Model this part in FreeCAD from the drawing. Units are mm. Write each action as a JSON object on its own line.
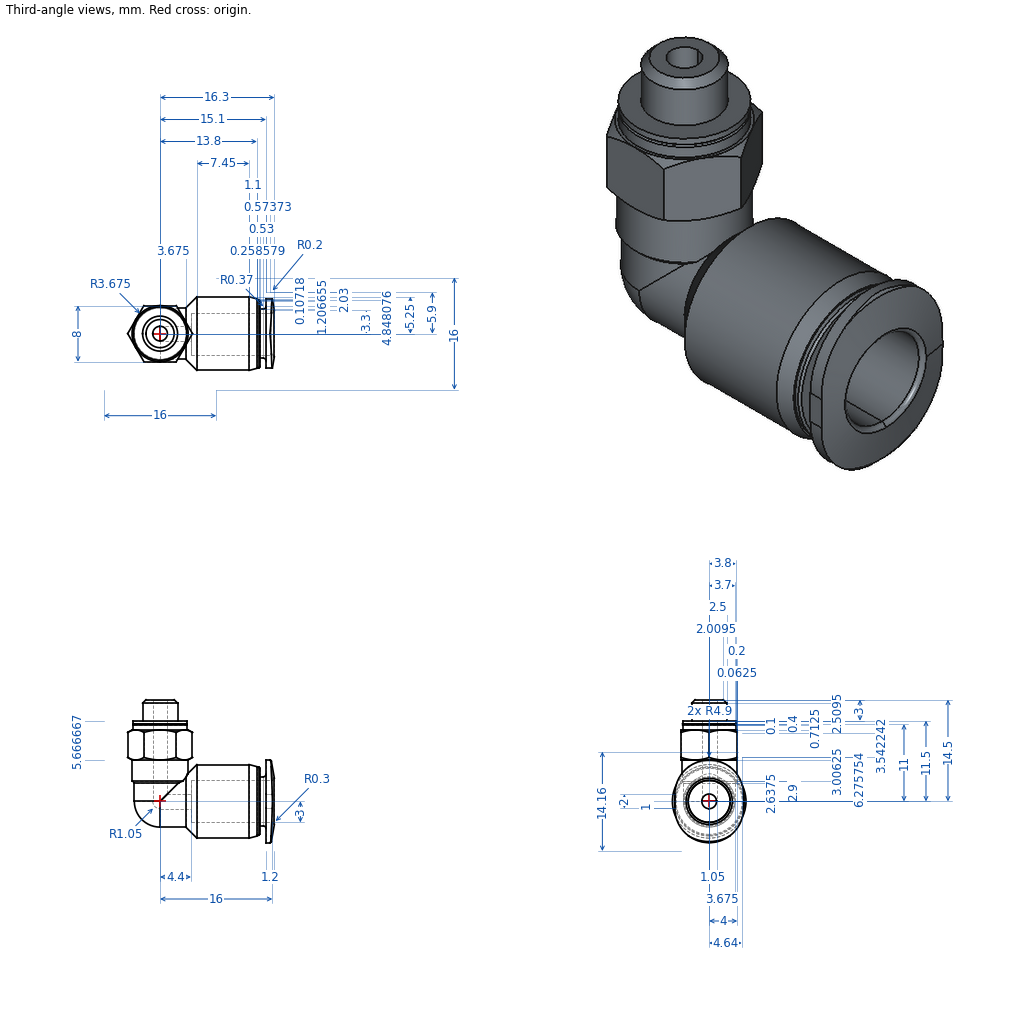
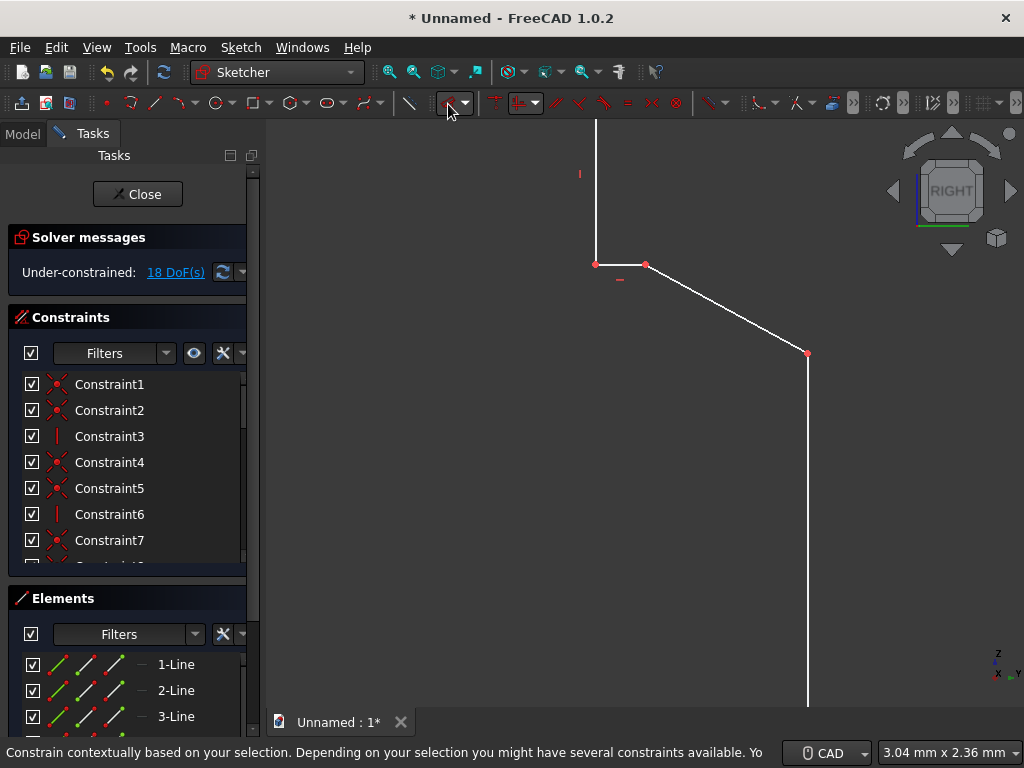
{"action": "scroll", "coordinate": [631, 265], "scroll_direction": "down", "scroll_amount": 10}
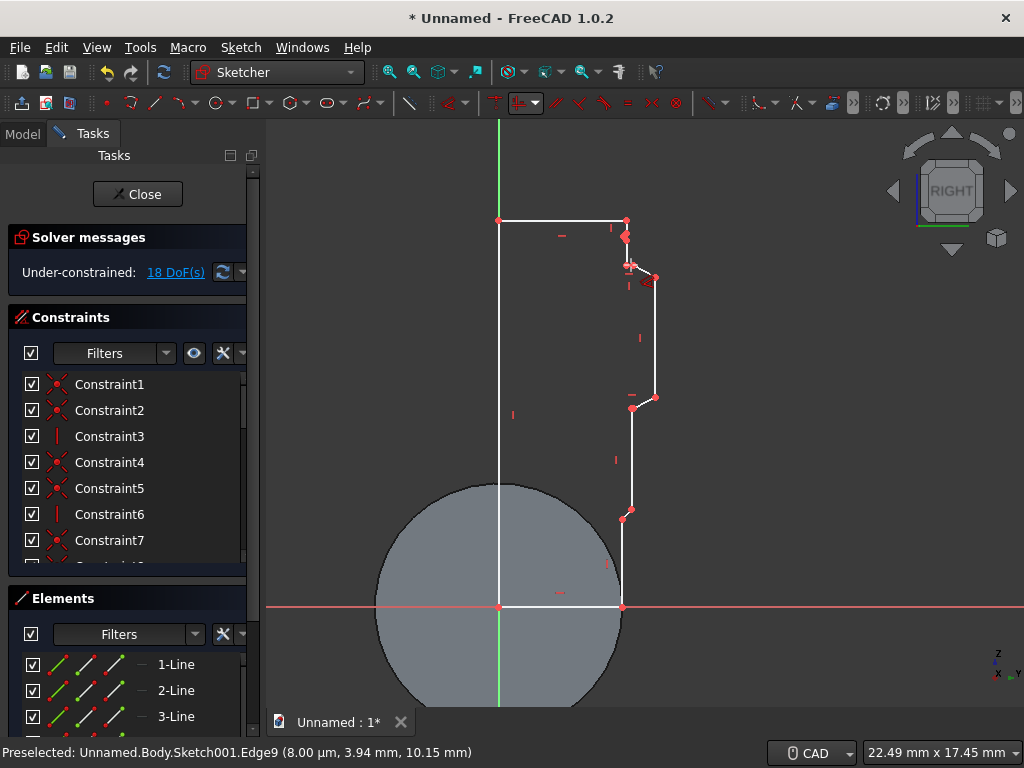
{"action": "scroll", "coordinate": [633, 409], "scroll_direction": "up", "scroll_amount": 10}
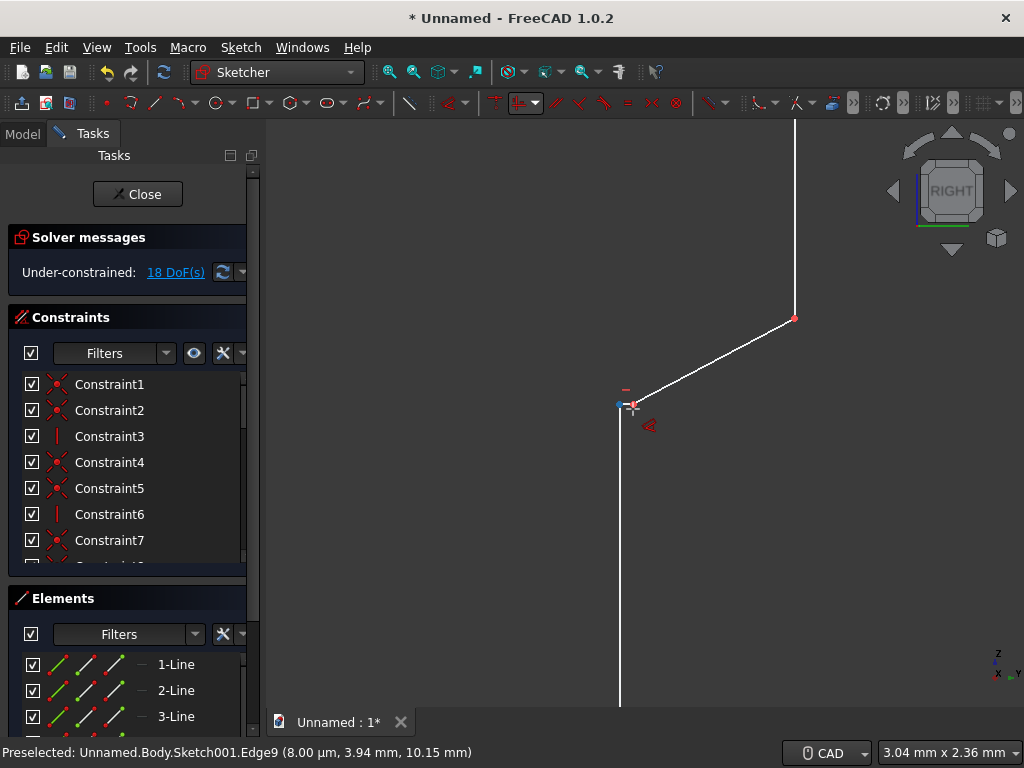
{"action": "left_click", "coordinate": [633, 404]}
{"action": "left_click", "coordinate": [464, 370]}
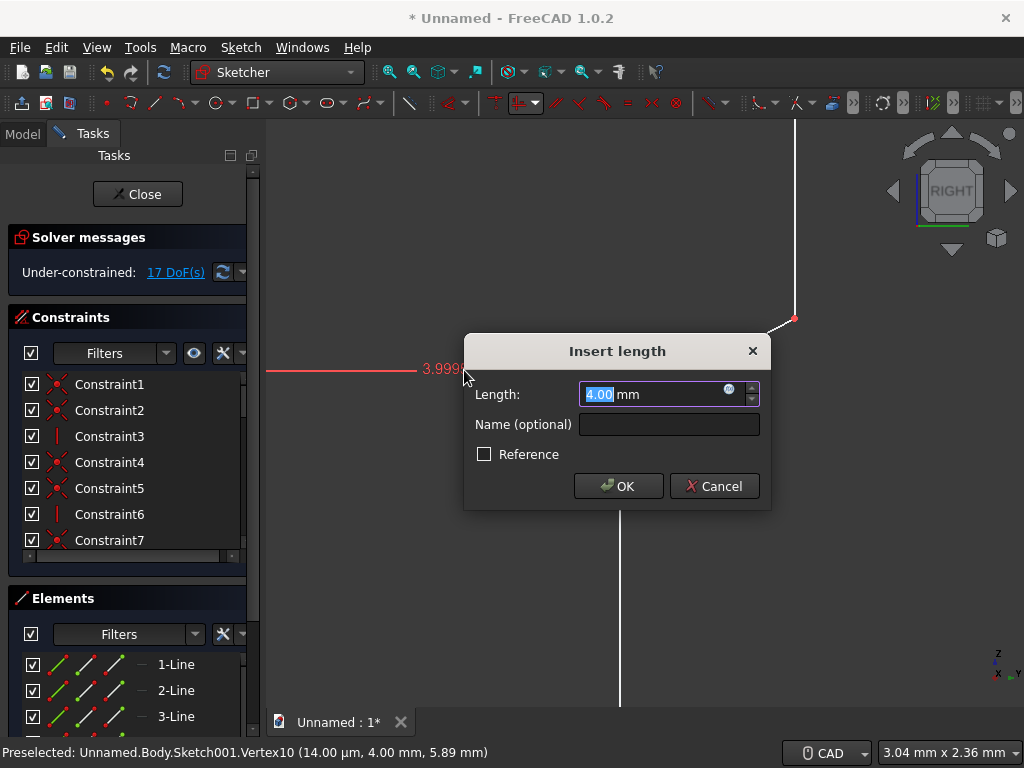
{"action": "type", "text": "4"}
{"action": "key", "text": "Return"}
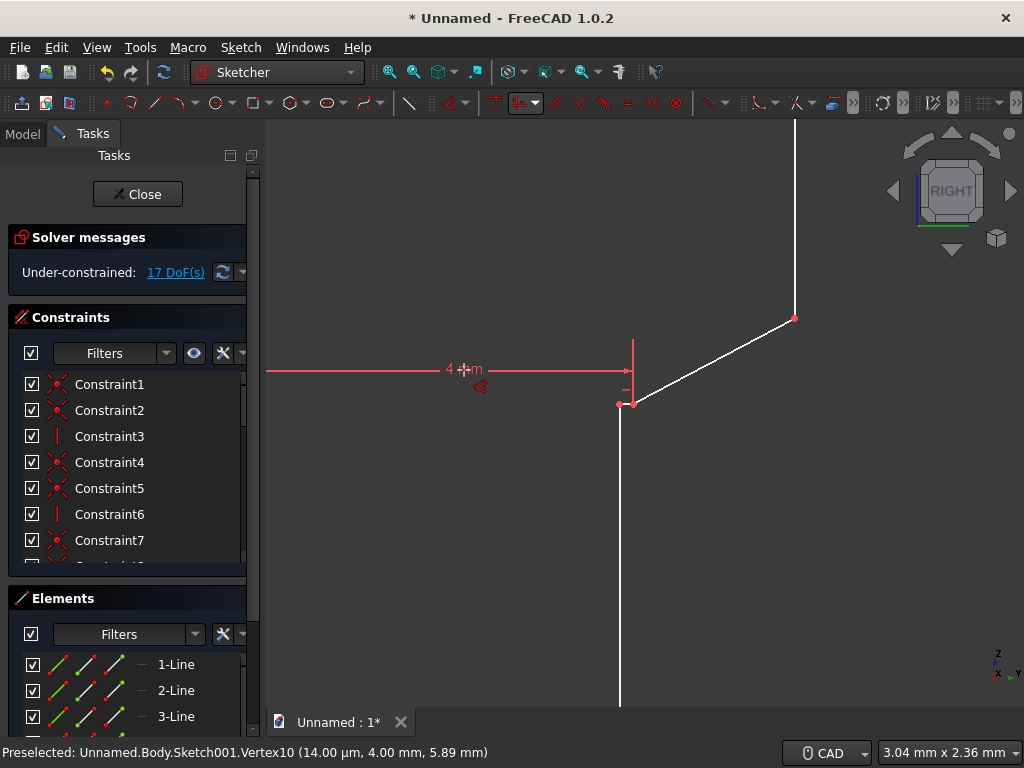
{"action": "scroll", "coordinate": [633, 409], "scroll_direction": "down", "scroll_amount": 10}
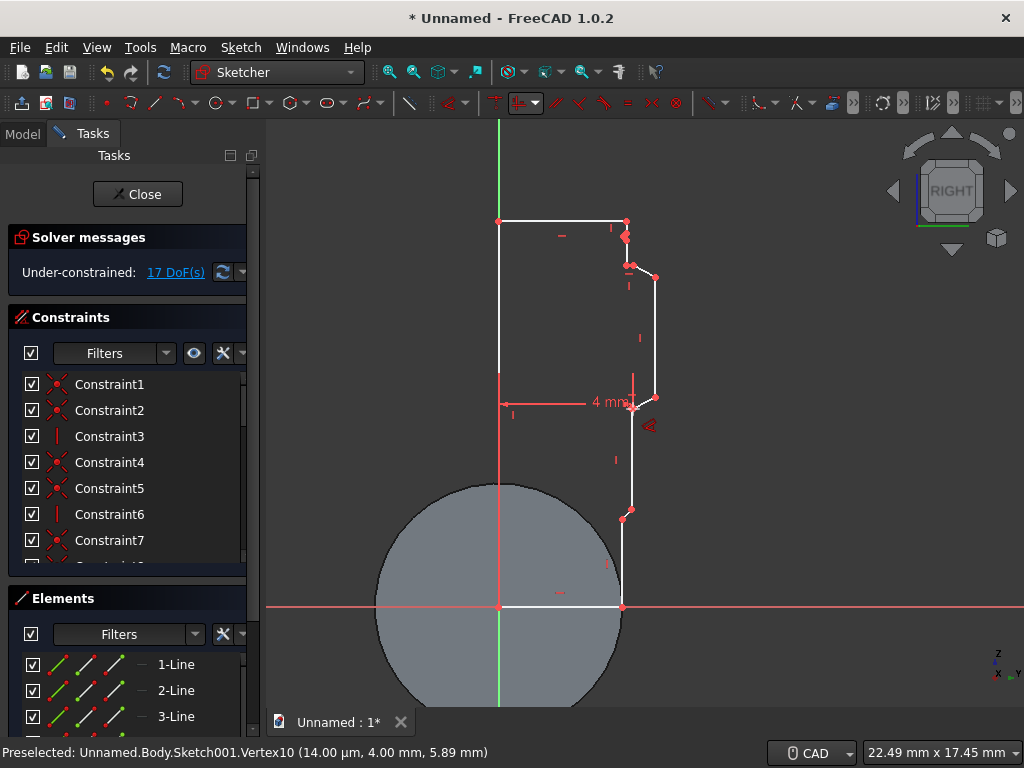
{"action": "scroll", "coordinate": [633, 265], "scroll_direction": "up", "scroll_amount": 4}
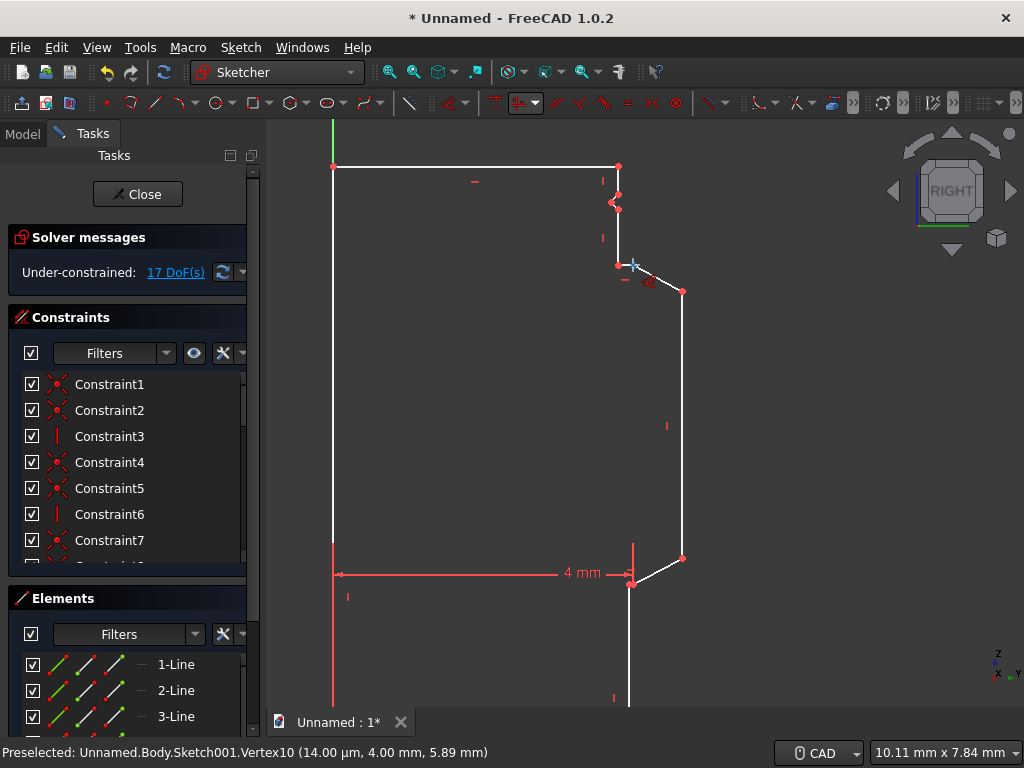
{"action": "left_click", "coordinate": [633, 265]}
{"action": "left_click", "coordinate": [483, 231]}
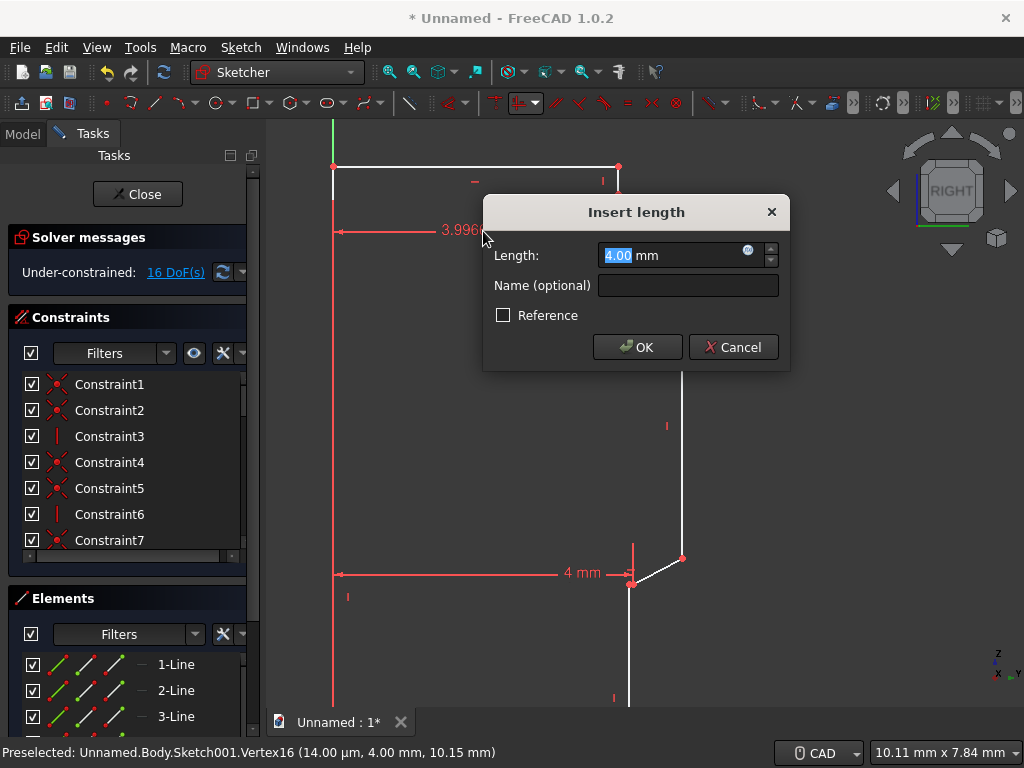
{"action": "type", "text": "4"}
{"action": "key", "text": "Return"}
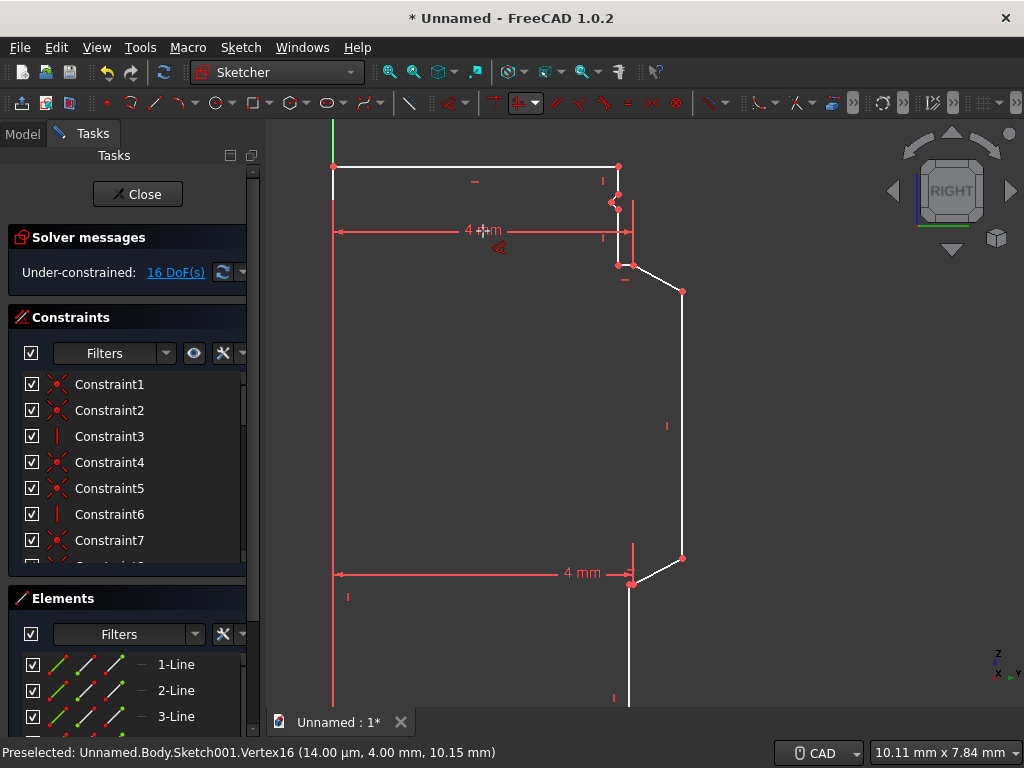
{"action": "scroll", "coordinate": [626, 265], "scroll_direction": "up", "scroll_amount": 5}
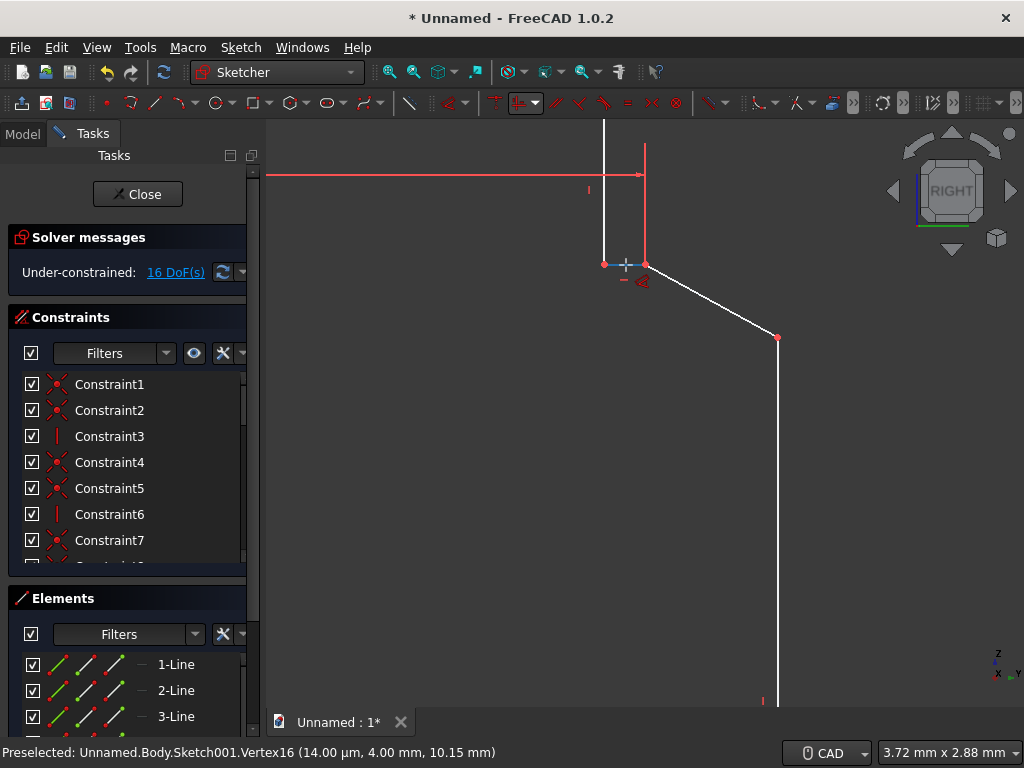
{"action": "left_click", "coordinate": [625, 265]}
{"action": "left_click", "coordinate": [625, 231]}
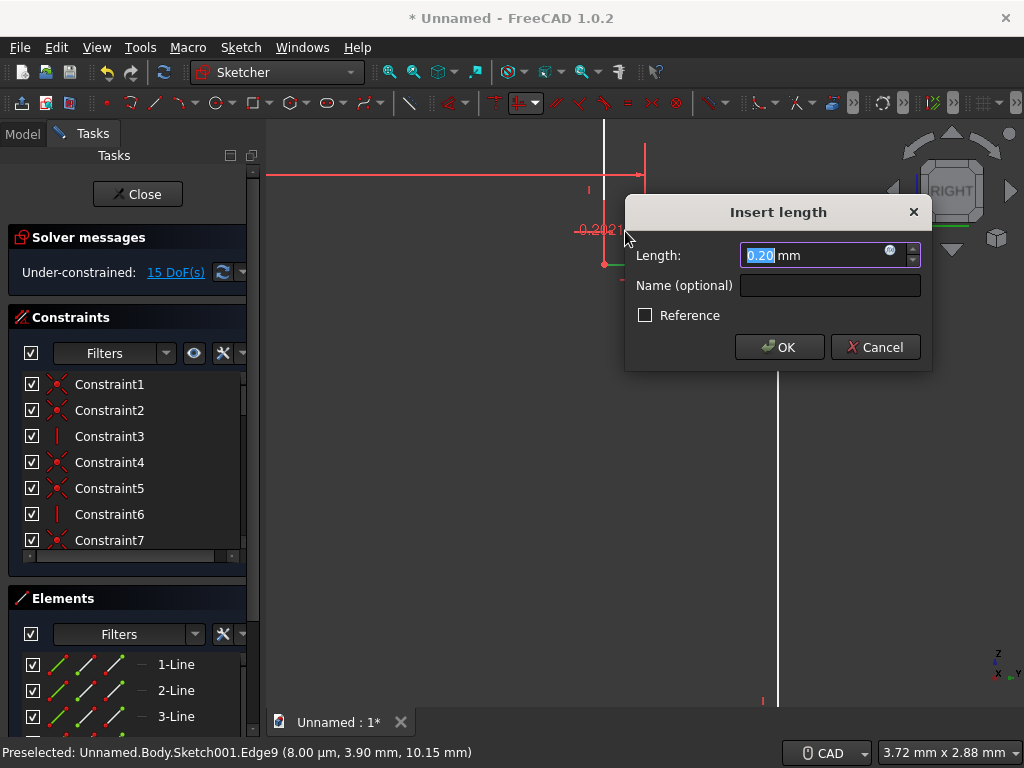
{"action": "type", "text": "0.2"}
{"action": "key", "text": "Return"}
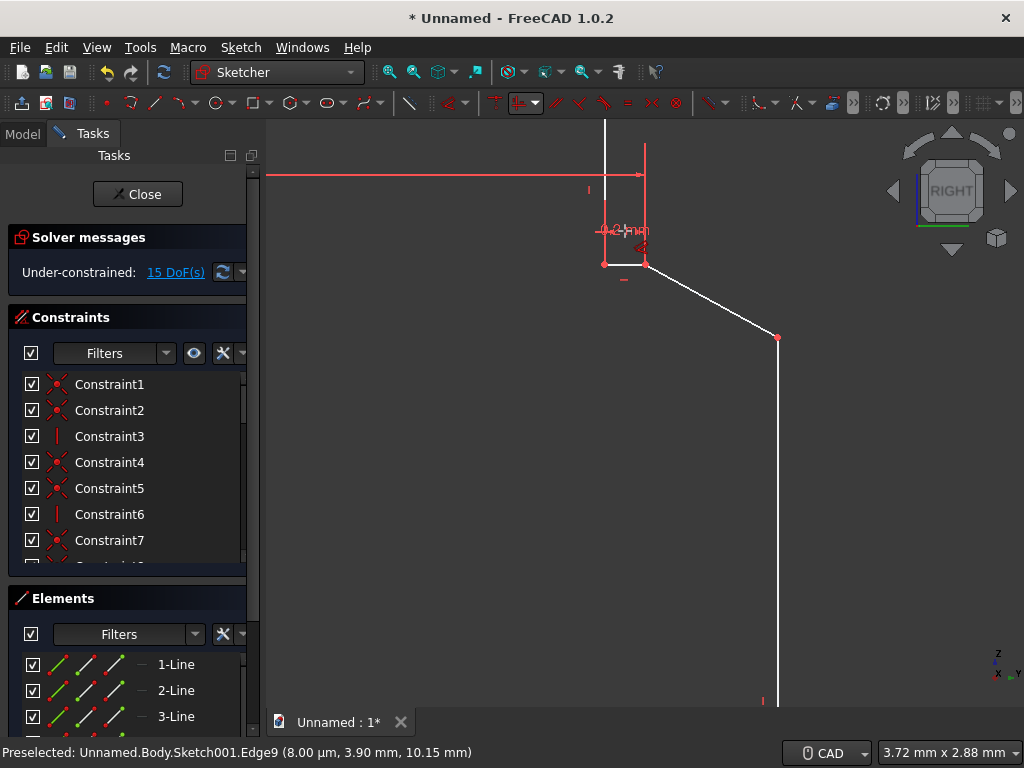
{"action": "scroll", "coordinate": [631, 265], "scroll_direction": "down", "scroll_amount": 9}